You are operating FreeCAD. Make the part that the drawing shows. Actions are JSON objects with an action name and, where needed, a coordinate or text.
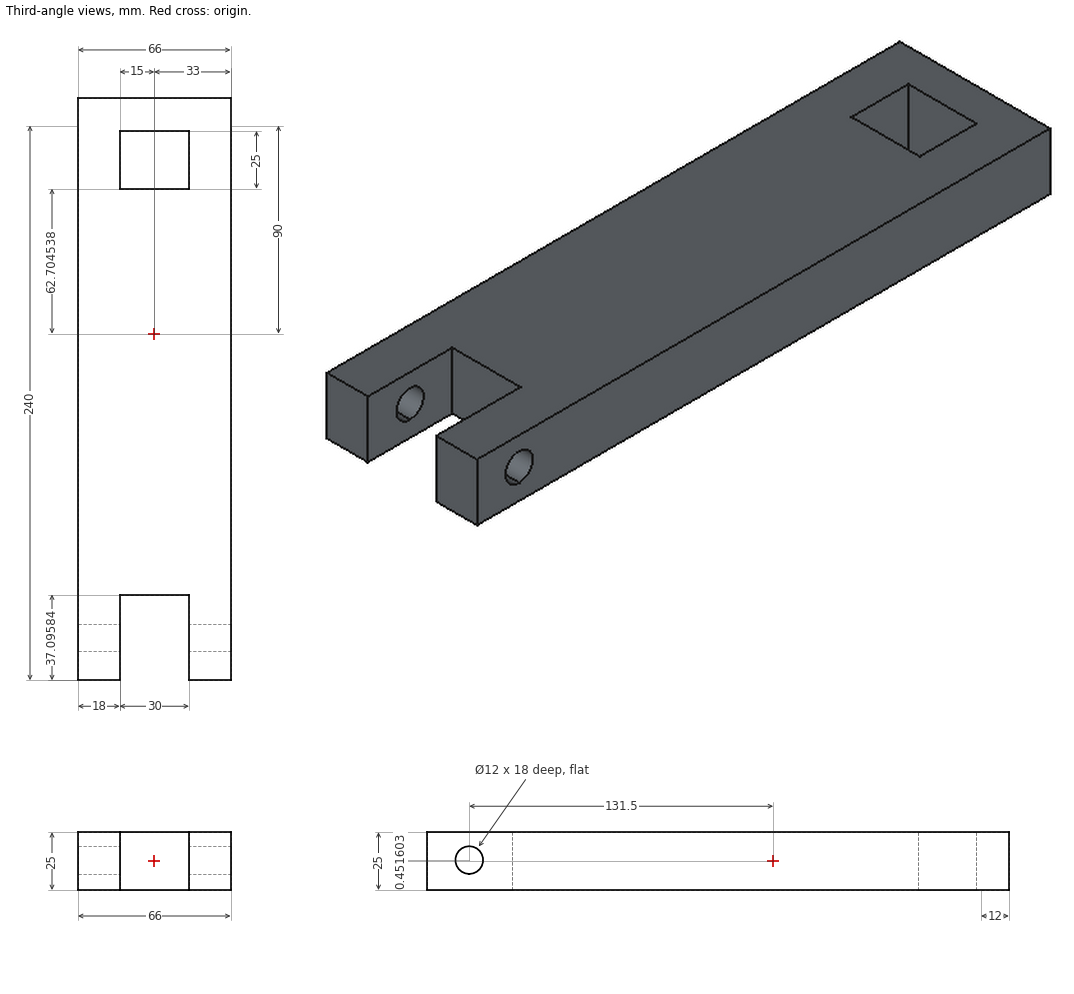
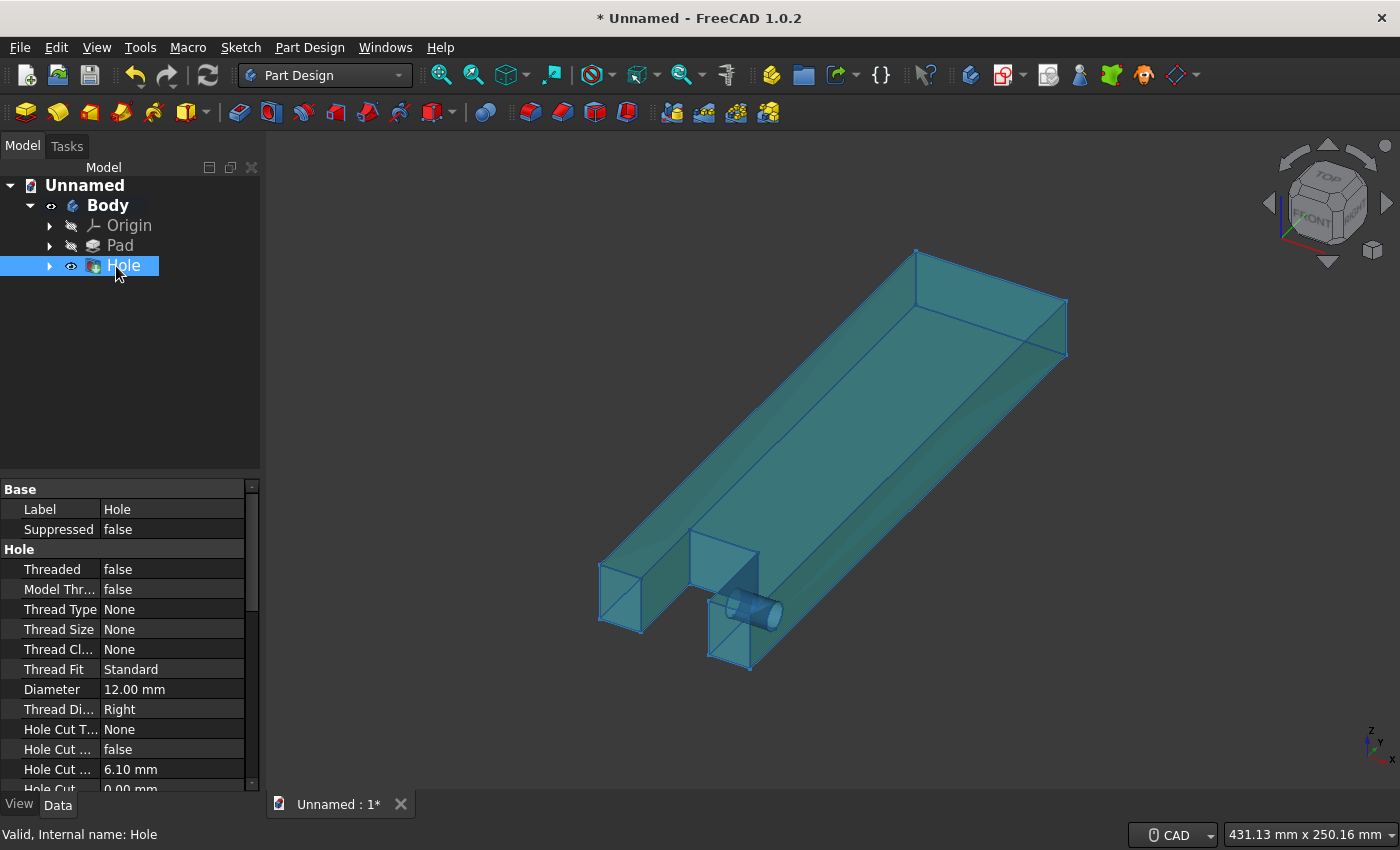
{"action": "left_click", "coordinate": [672, 112]}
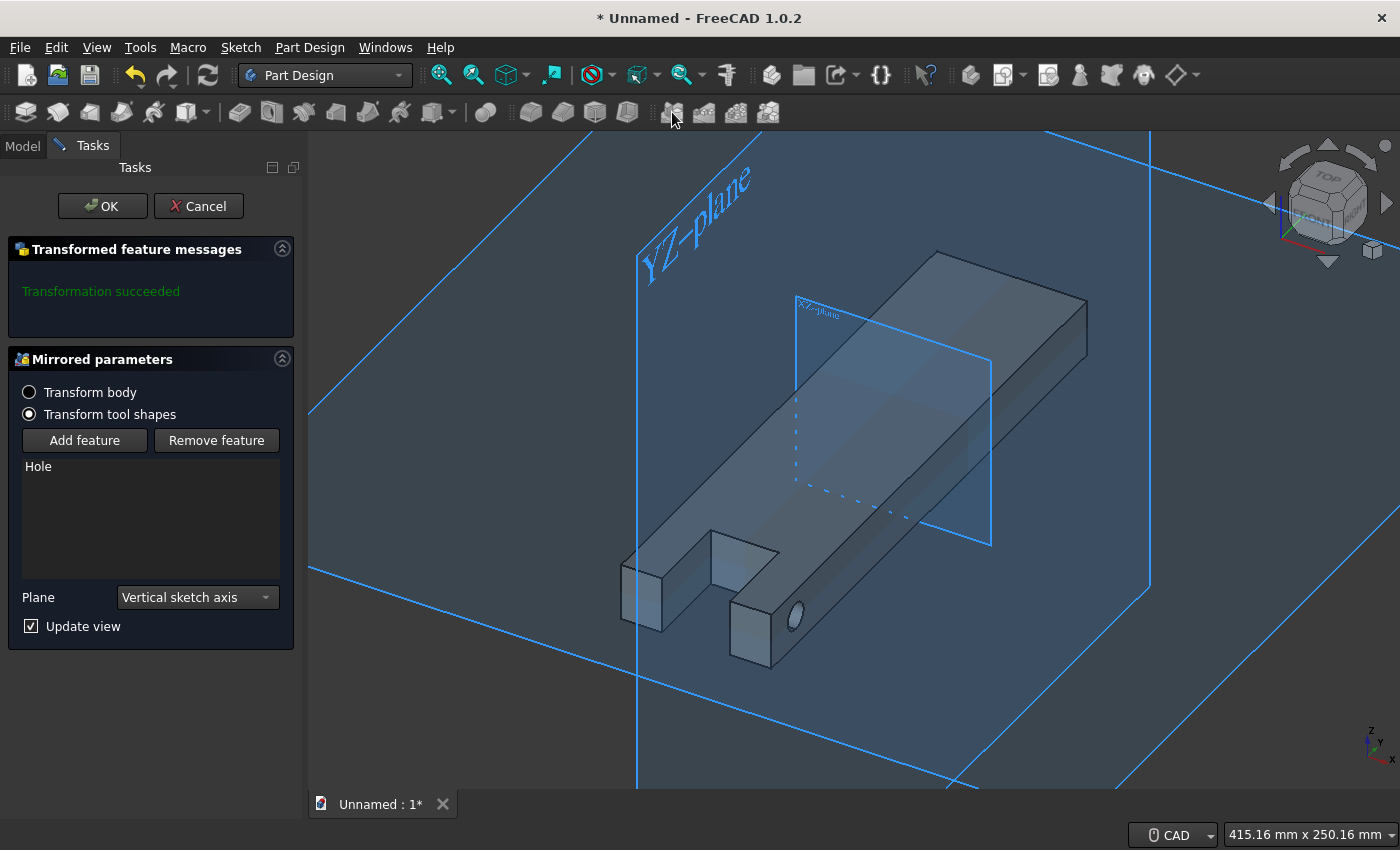
{"action": "left_click", "coordinate": [198, 598]}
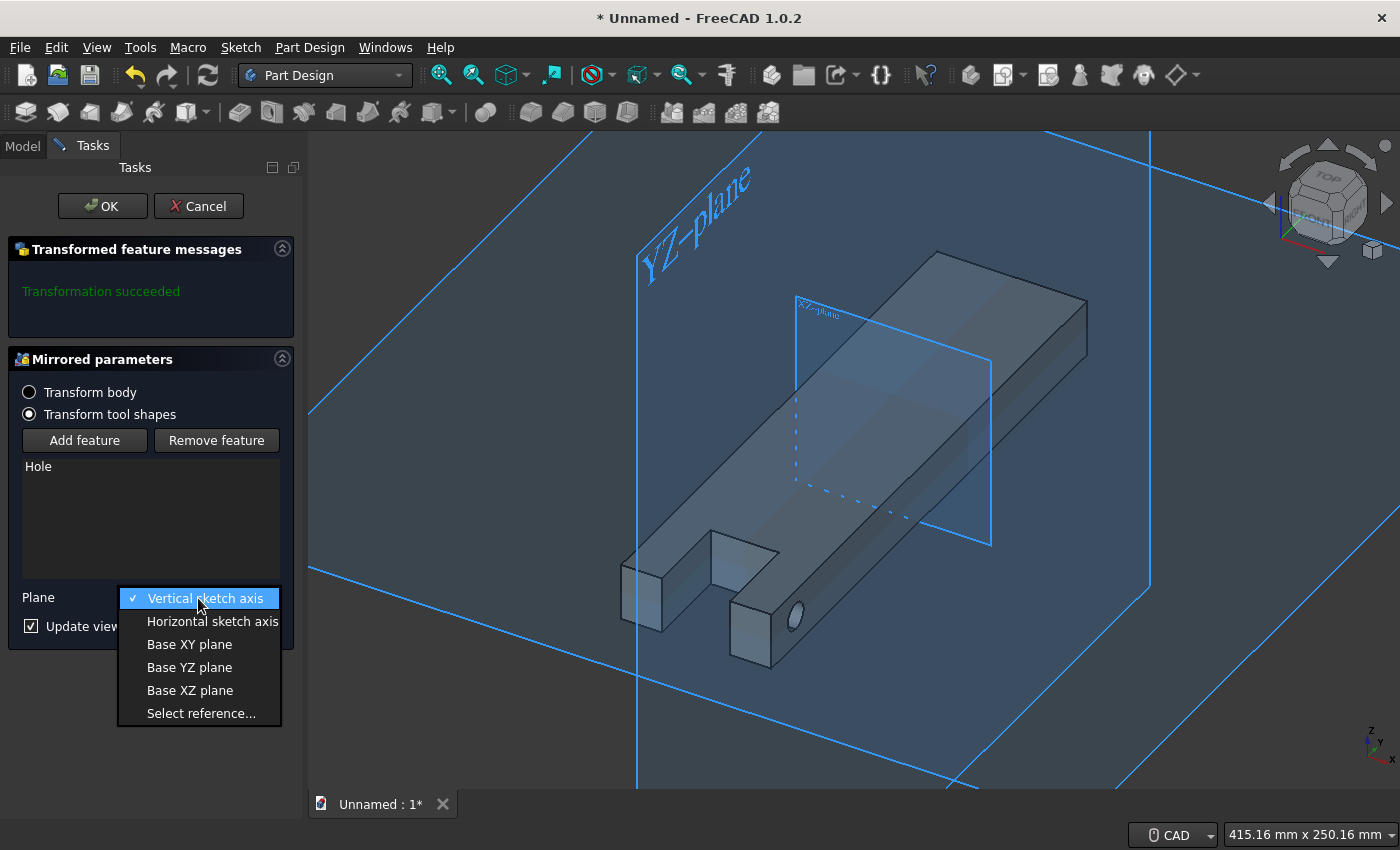
{"action": "left_click", "coordinate": [198, 668]}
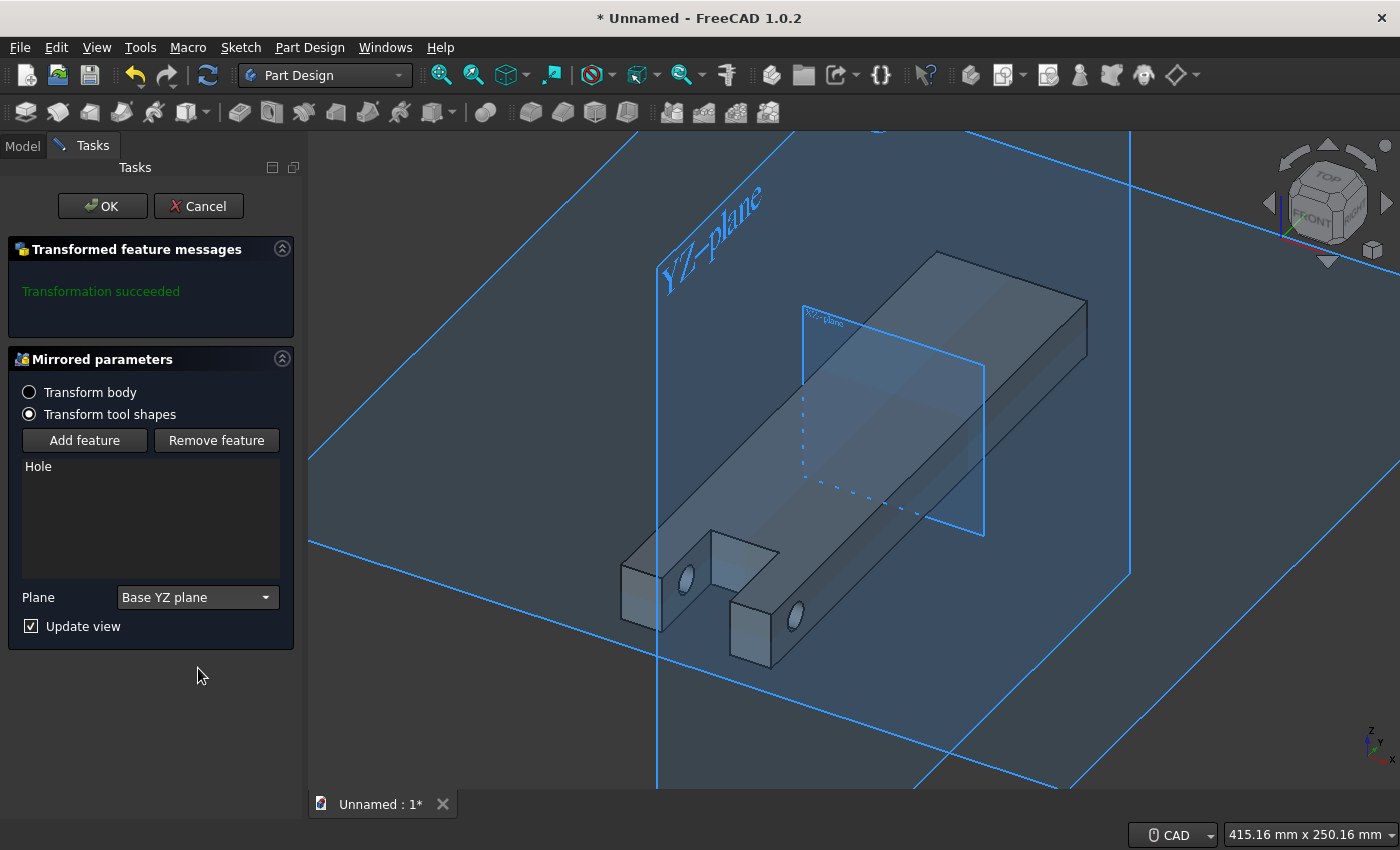
{"action": "left_click", "coordinate": [103, 206]}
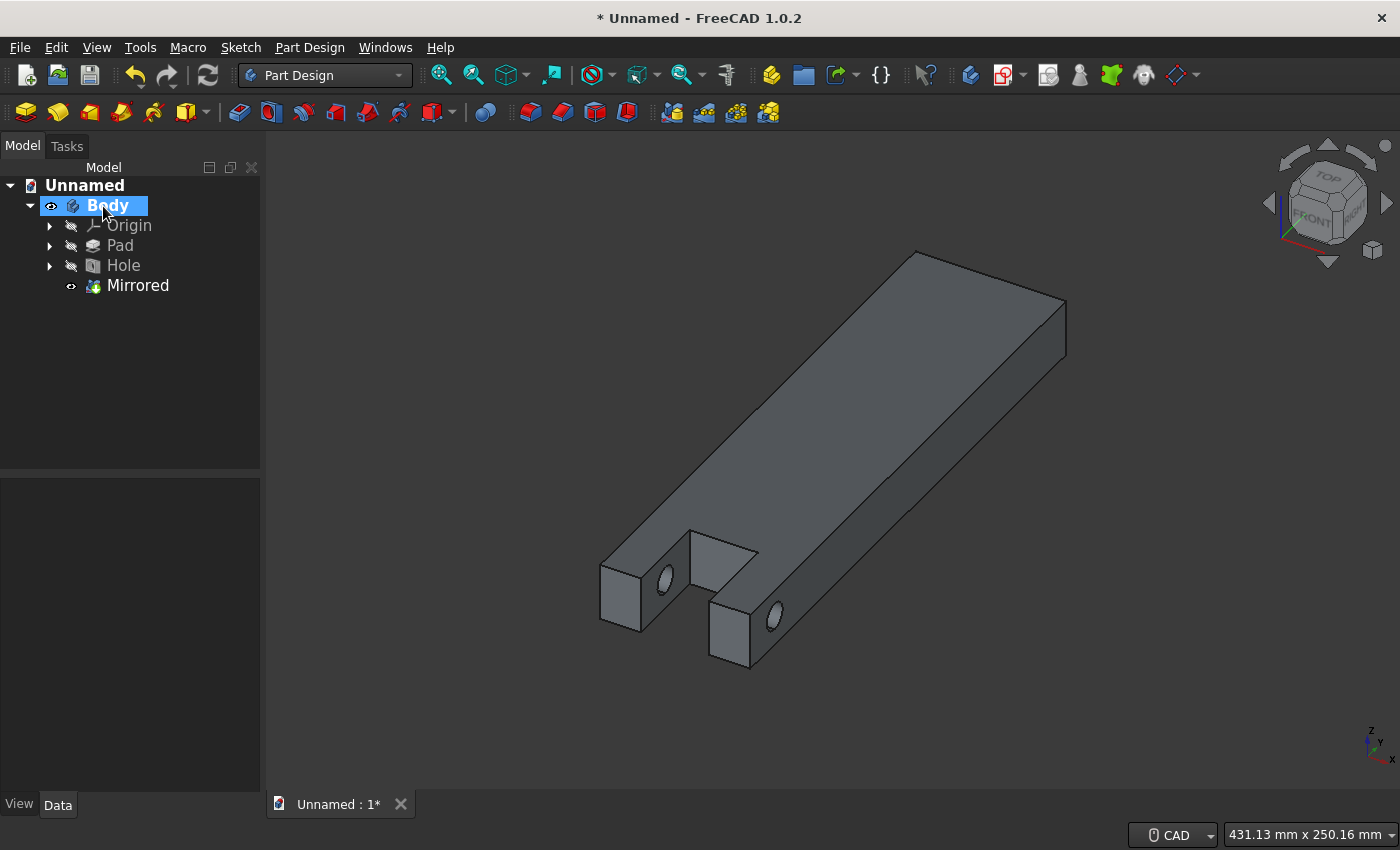
{"action": "key", "text": "4"}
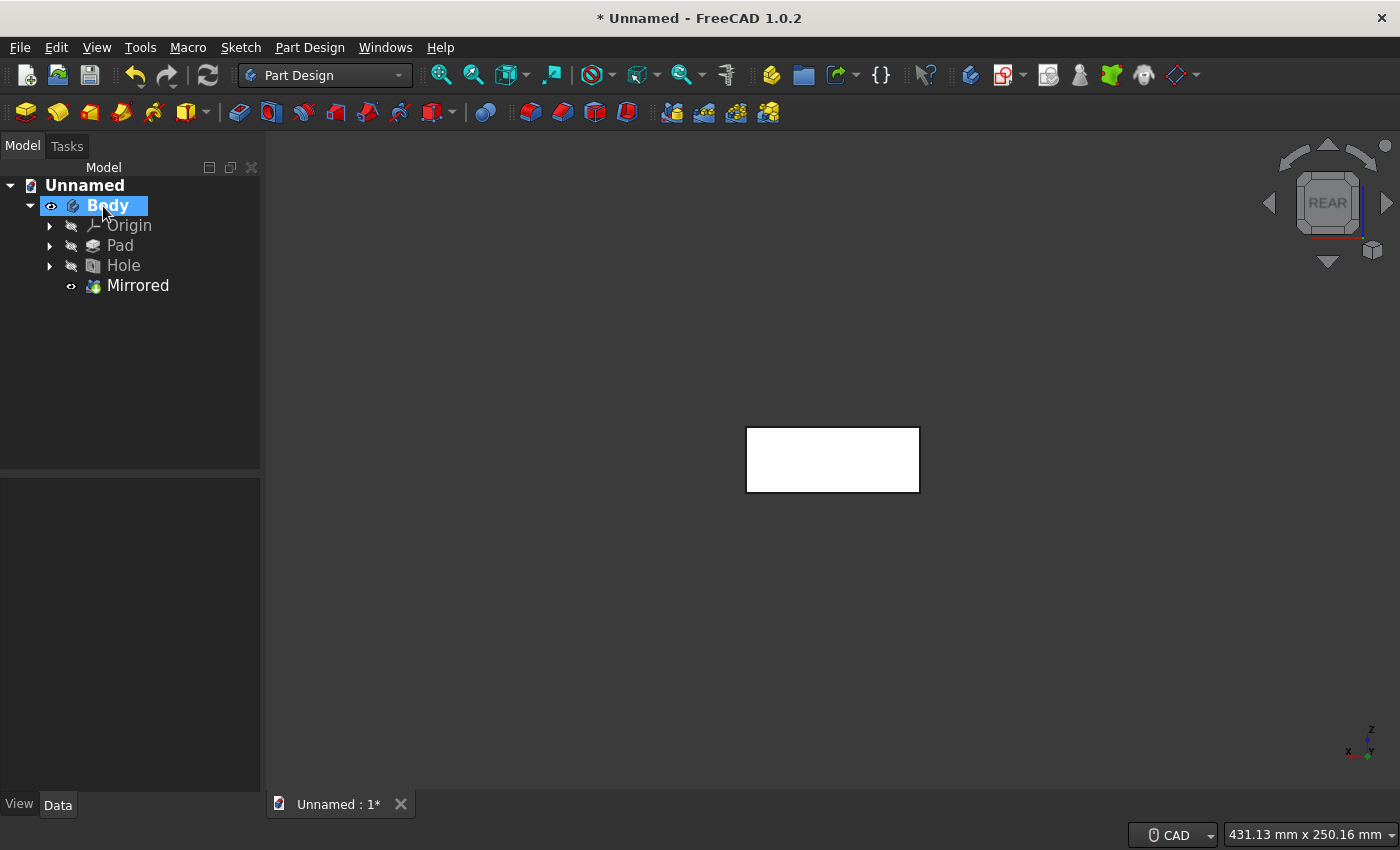
{"action": "left_click", "coordinate": [442, 76]}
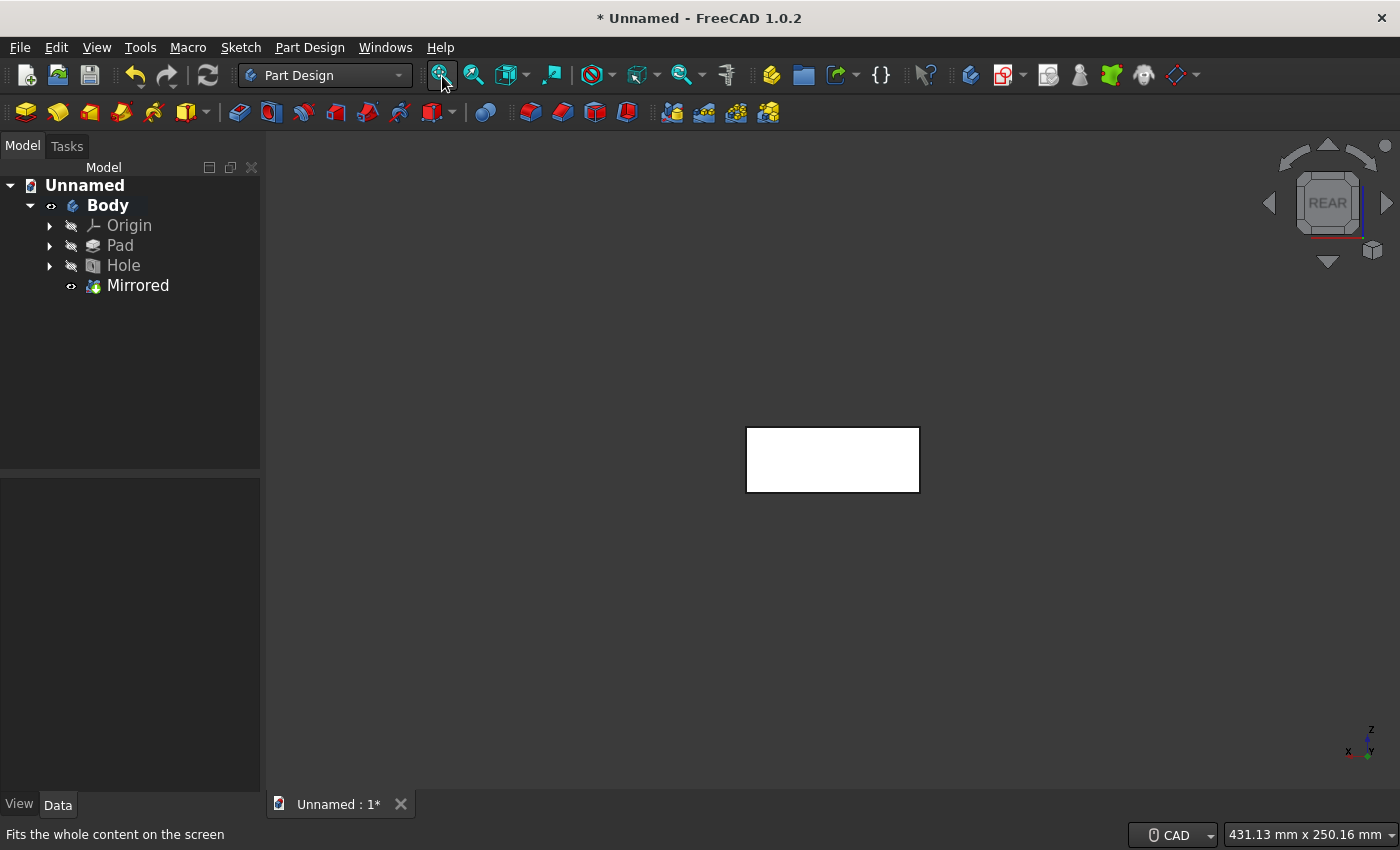
{"action": "left_click", "coordinate": [783, 459]}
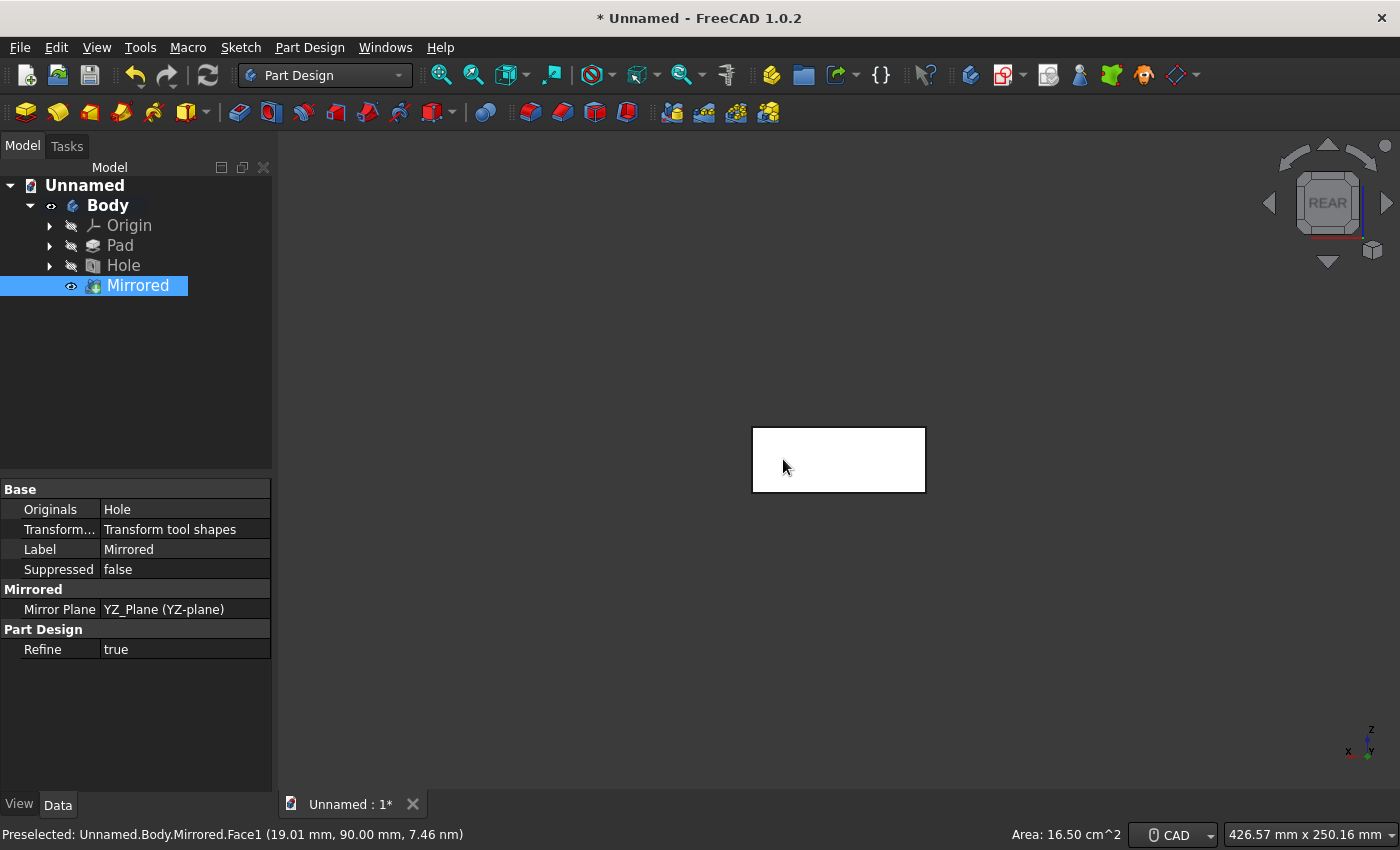
{"action": "left_click", "coordinate": [1004, 76]}